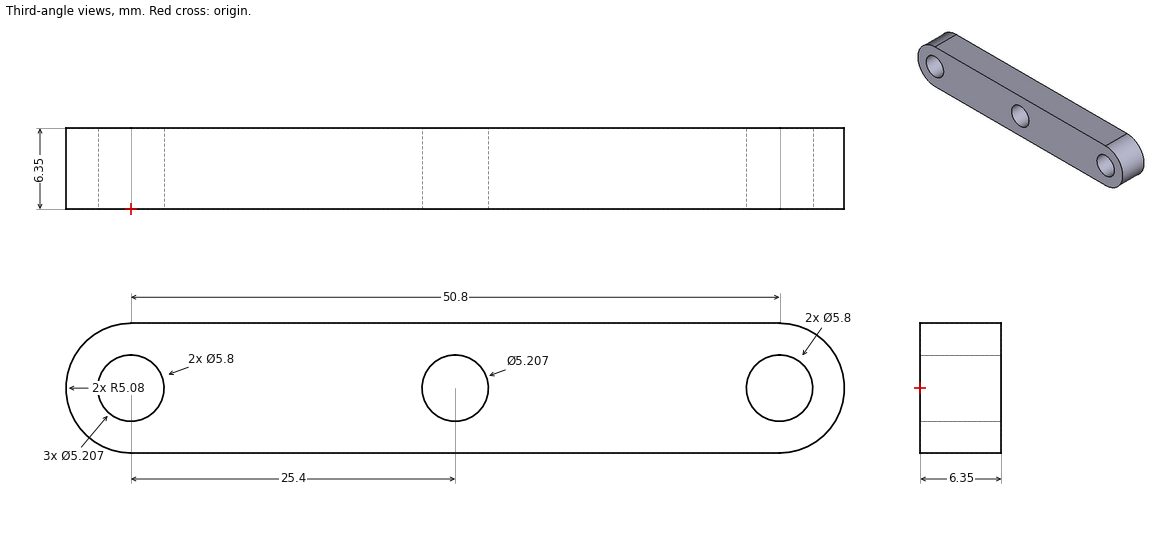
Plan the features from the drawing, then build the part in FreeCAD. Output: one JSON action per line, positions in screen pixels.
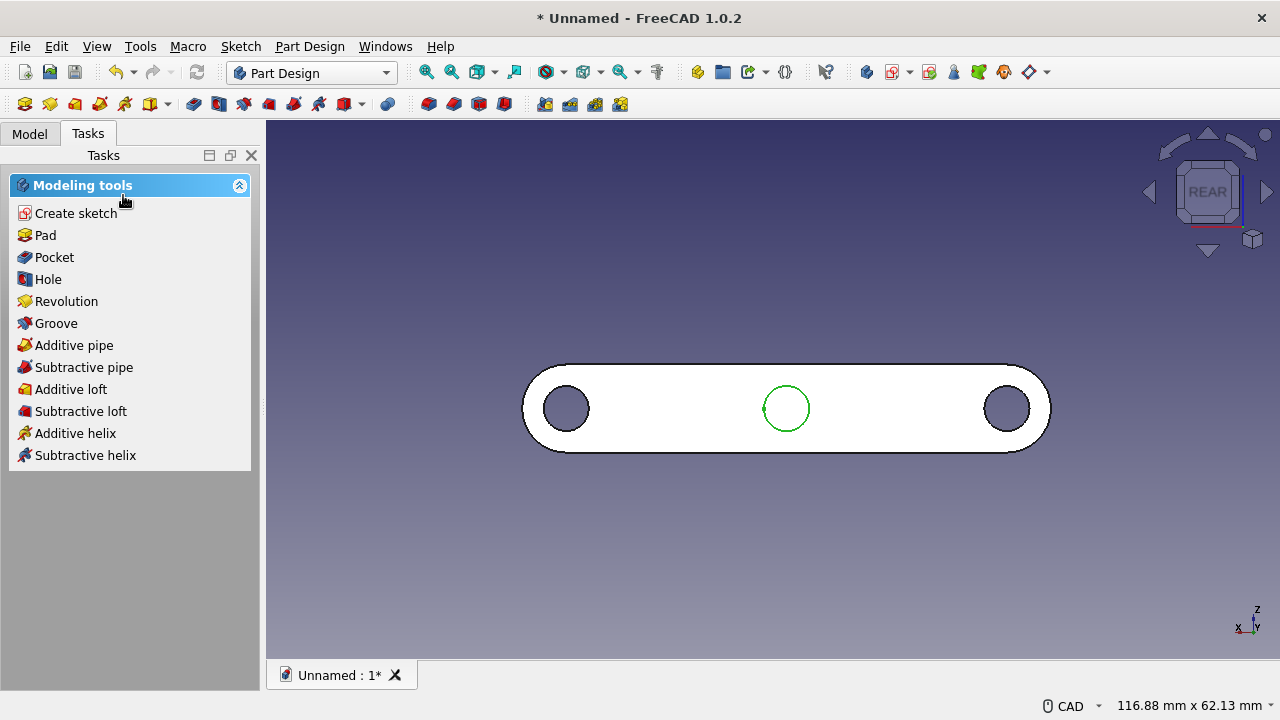
{"action": "left_click", "coordinate": [194, 104]}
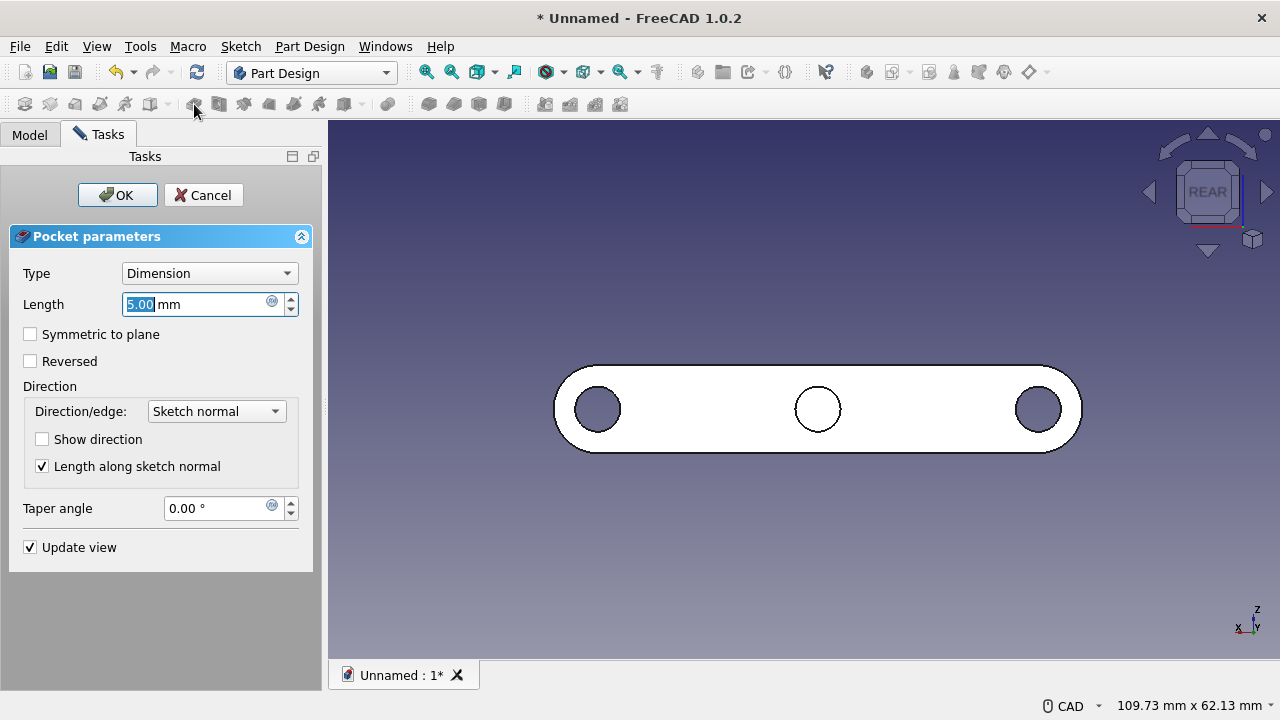
{"action": "left_click", "coordinate": [210, 274]}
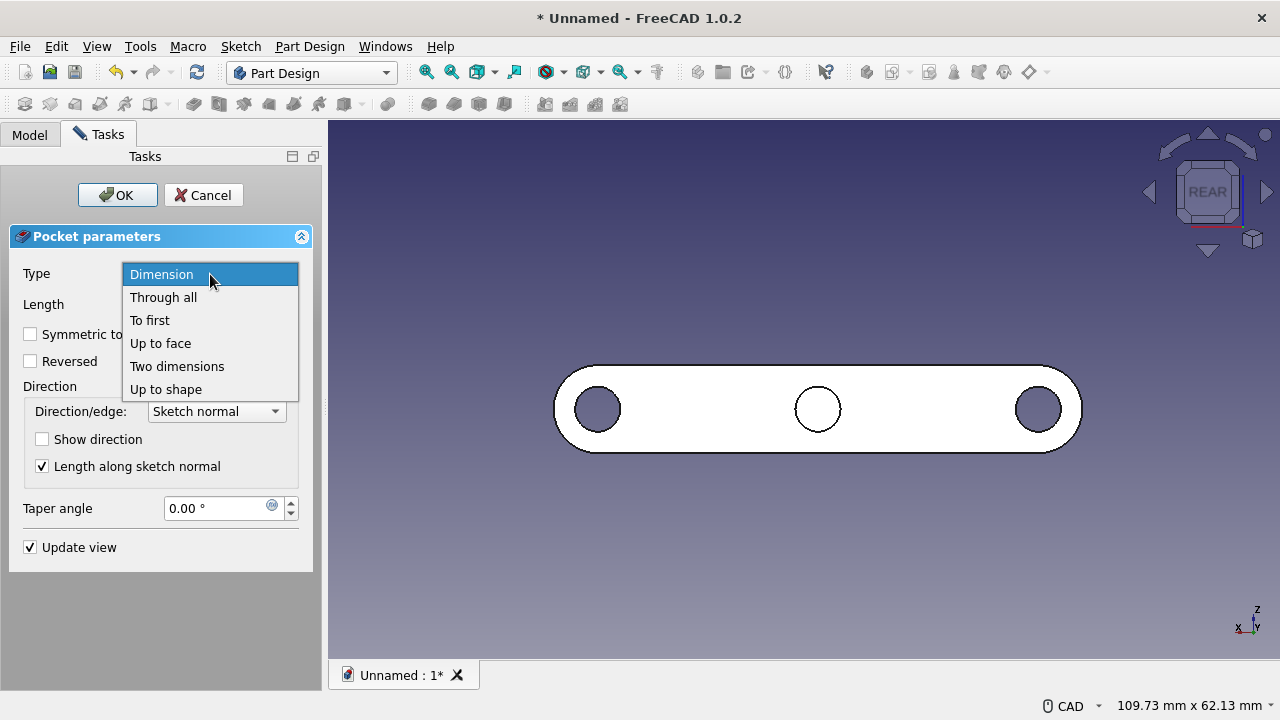
{"action": "left_click", "coordinate": [208, 298]}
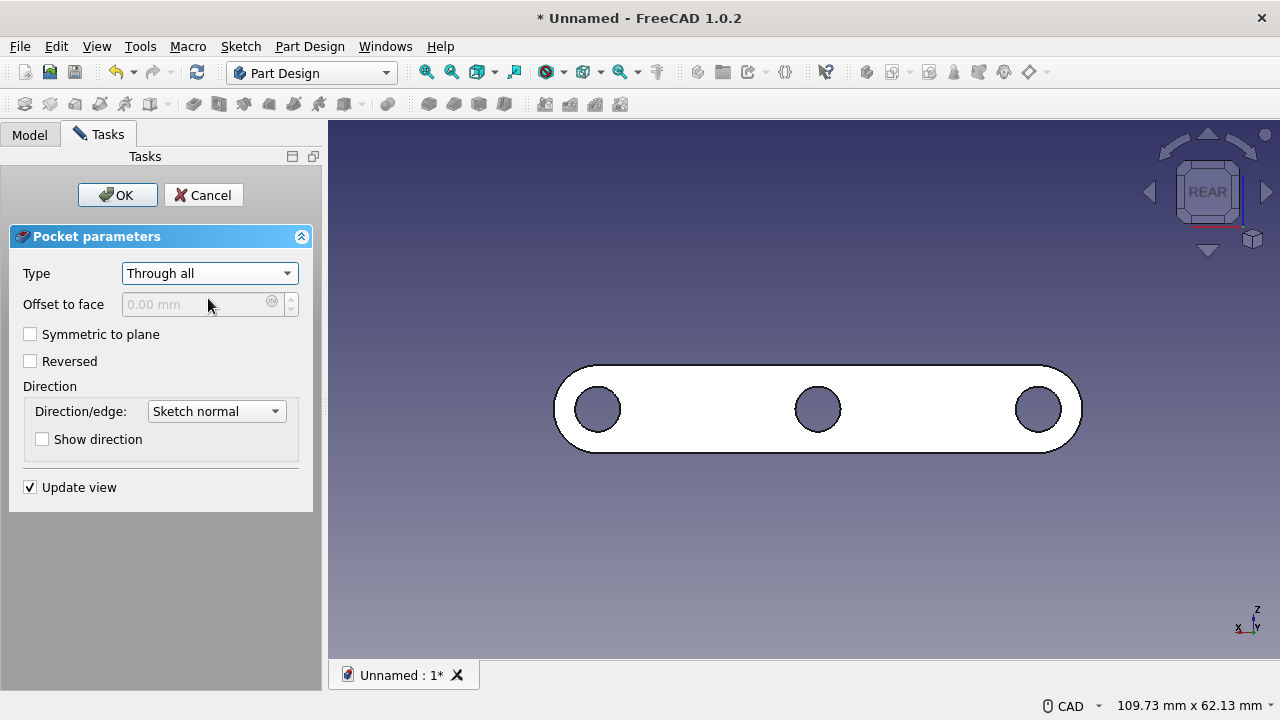
{"action": "left_click", "coordinate": [118, 195]}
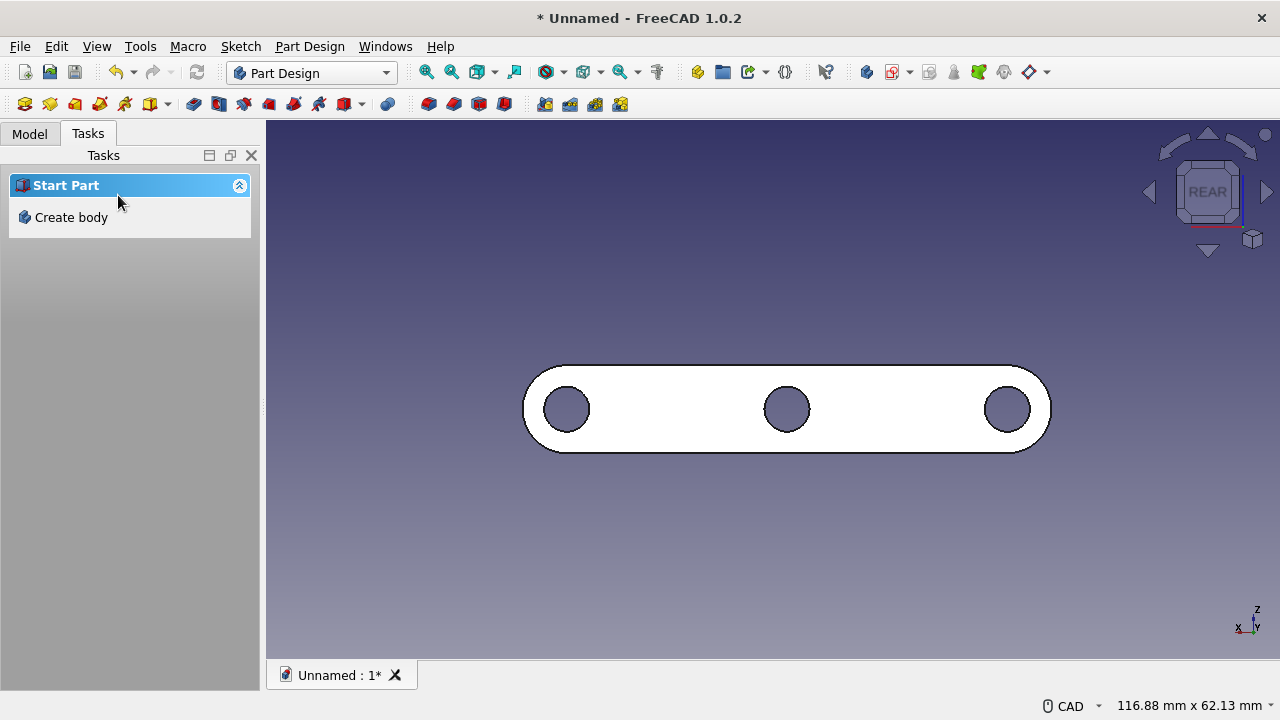
{"action": "key", "text": "0"}